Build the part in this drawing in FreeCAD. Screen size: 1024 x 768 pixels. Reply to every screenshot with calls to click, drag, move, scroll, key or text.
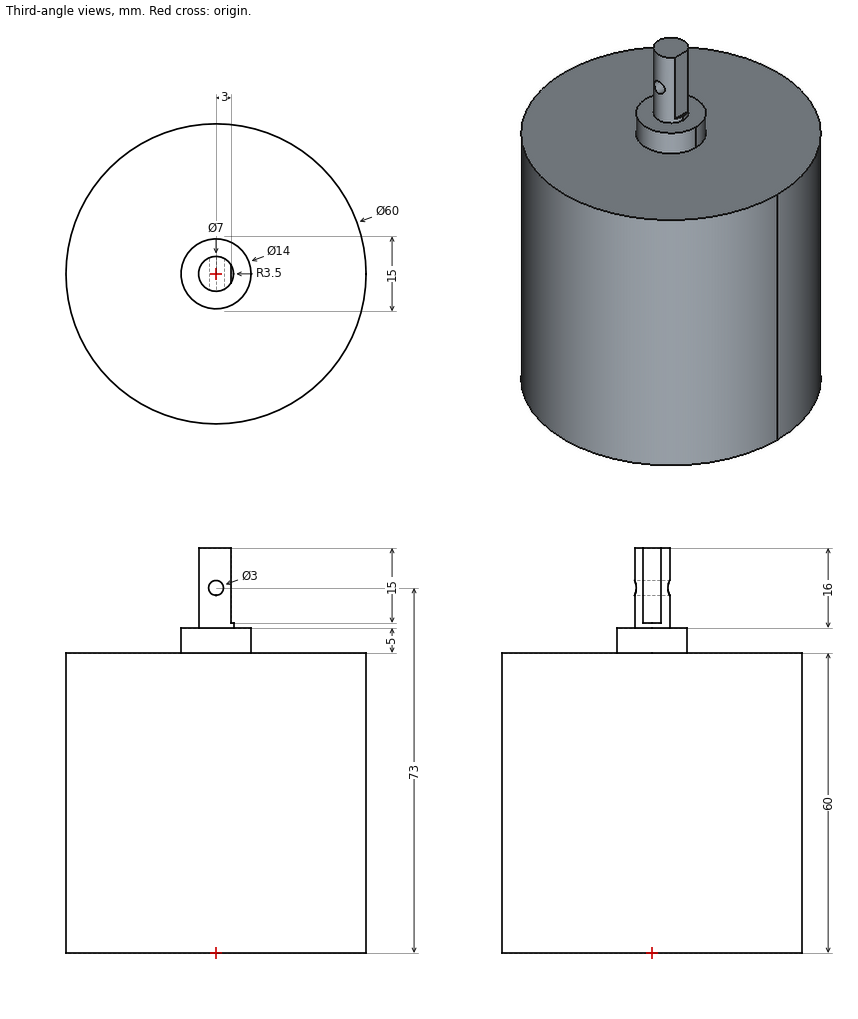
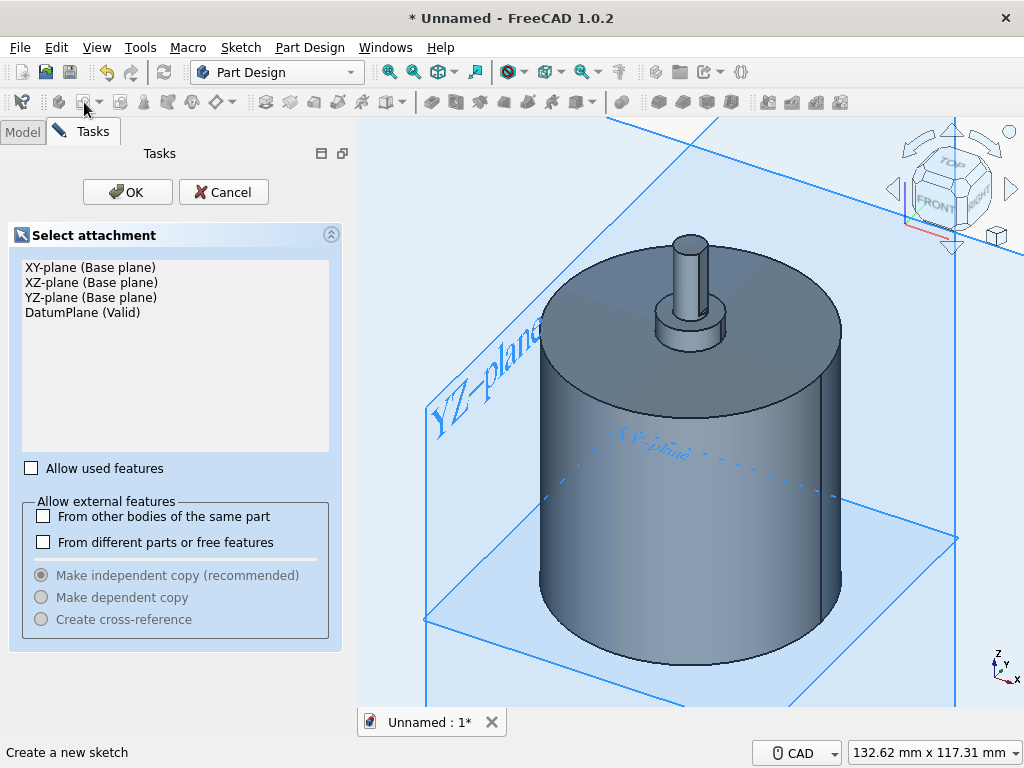
click(82, 282)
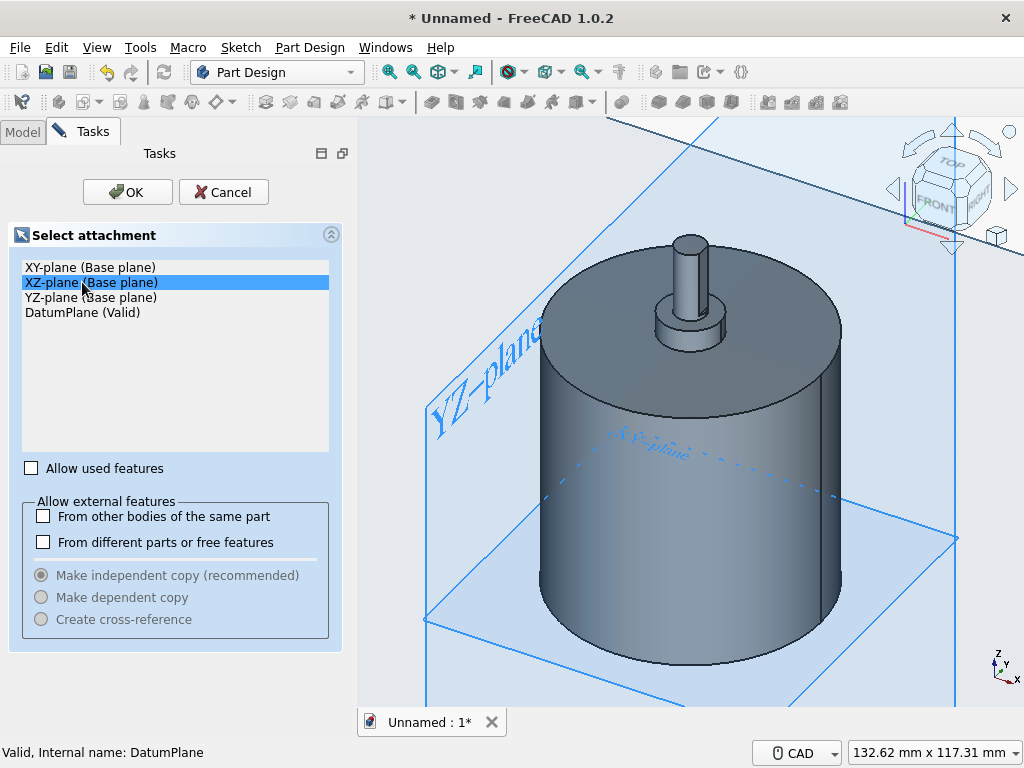
click(128, 192)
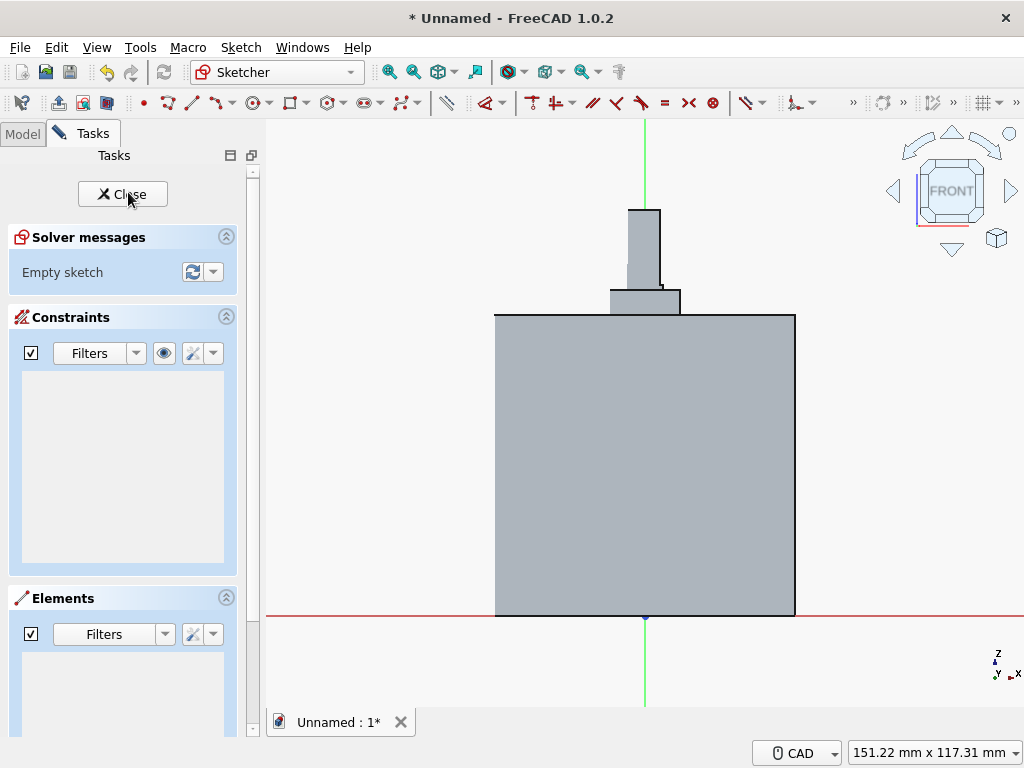
click(108, 104)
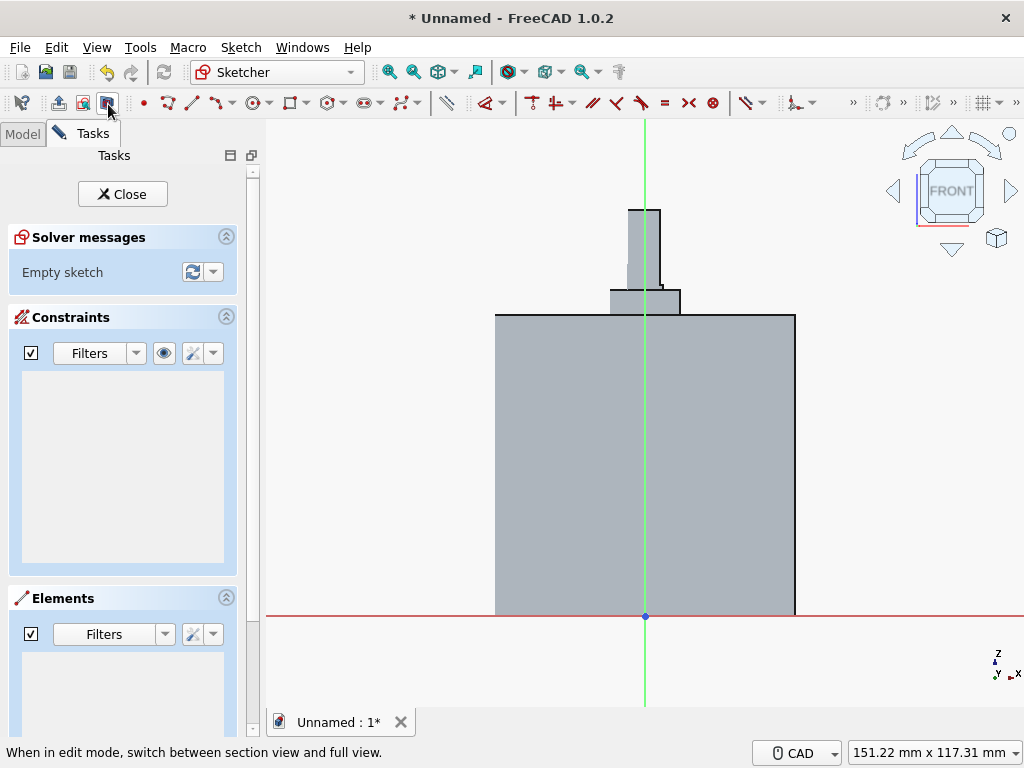
scroll(649, 242, up, 15)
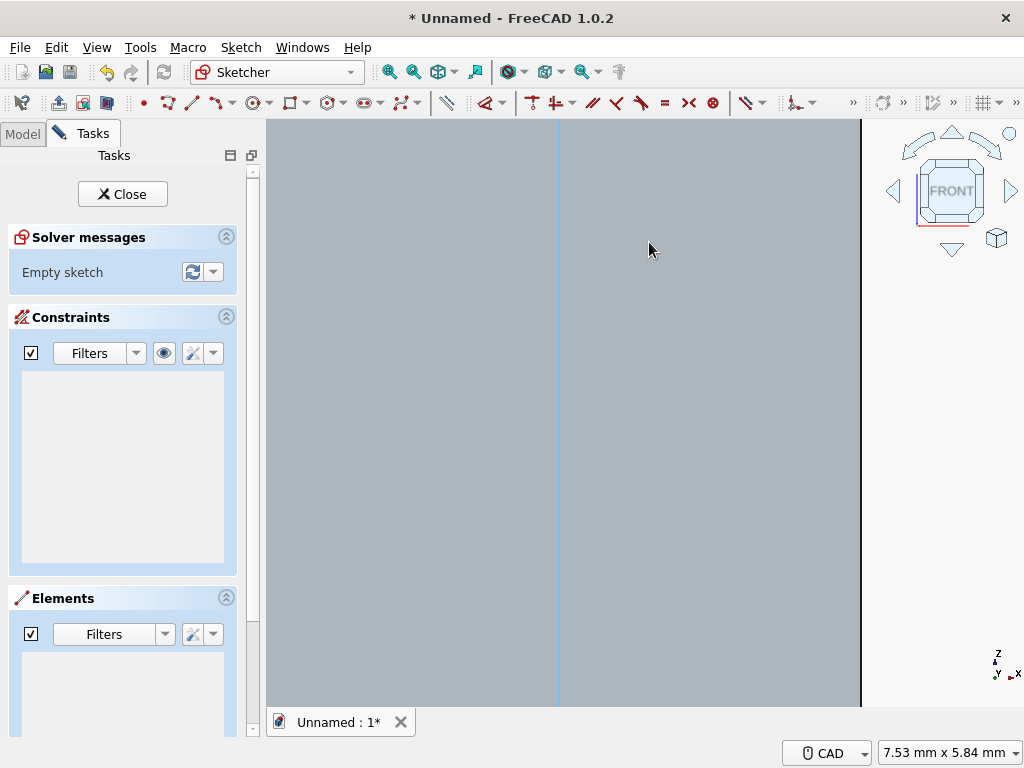
click(254, 104)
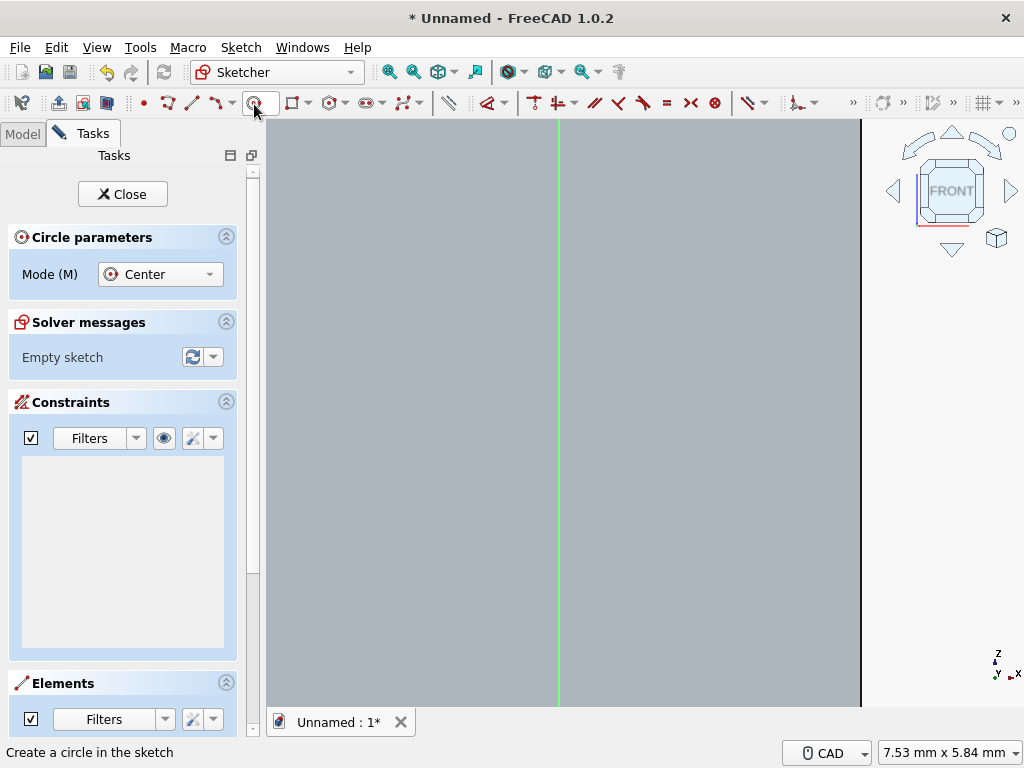
click(559, 401)
move(666, 294)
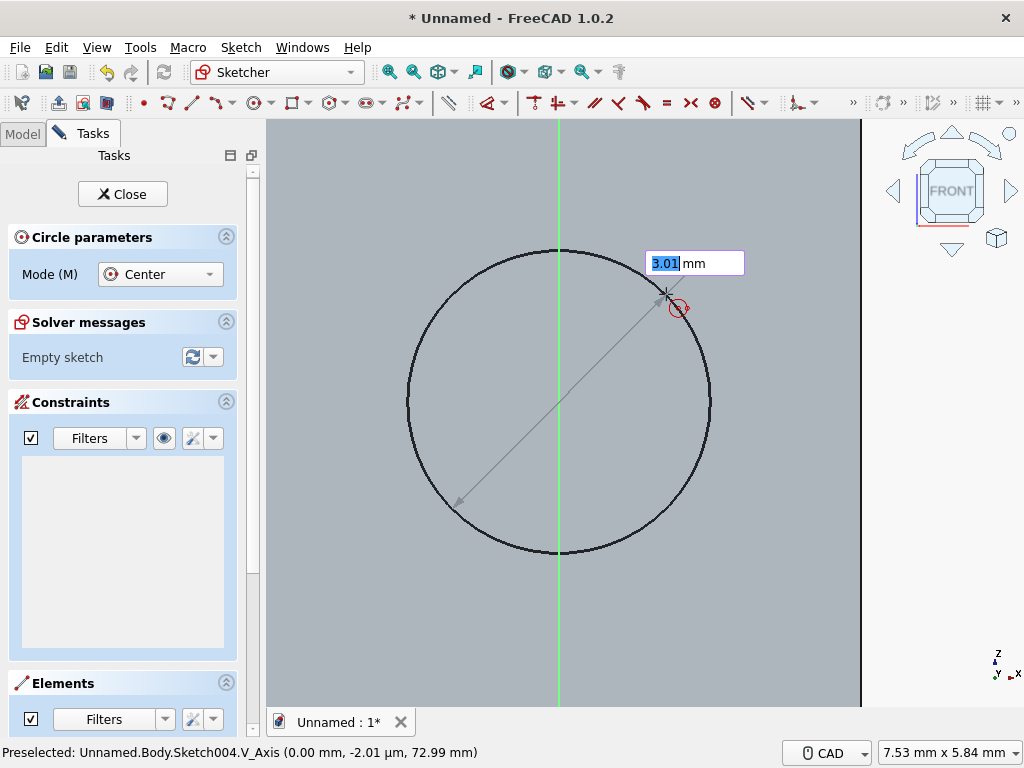
text(3)
key(Return)
key(Escape)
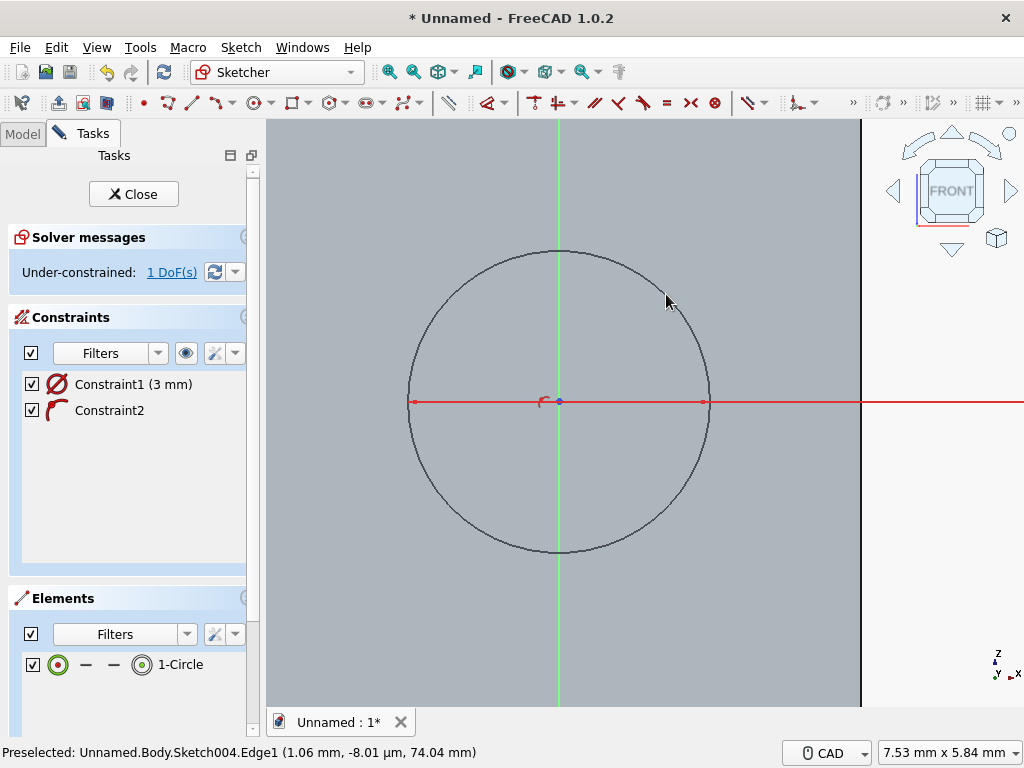
click(488, 104)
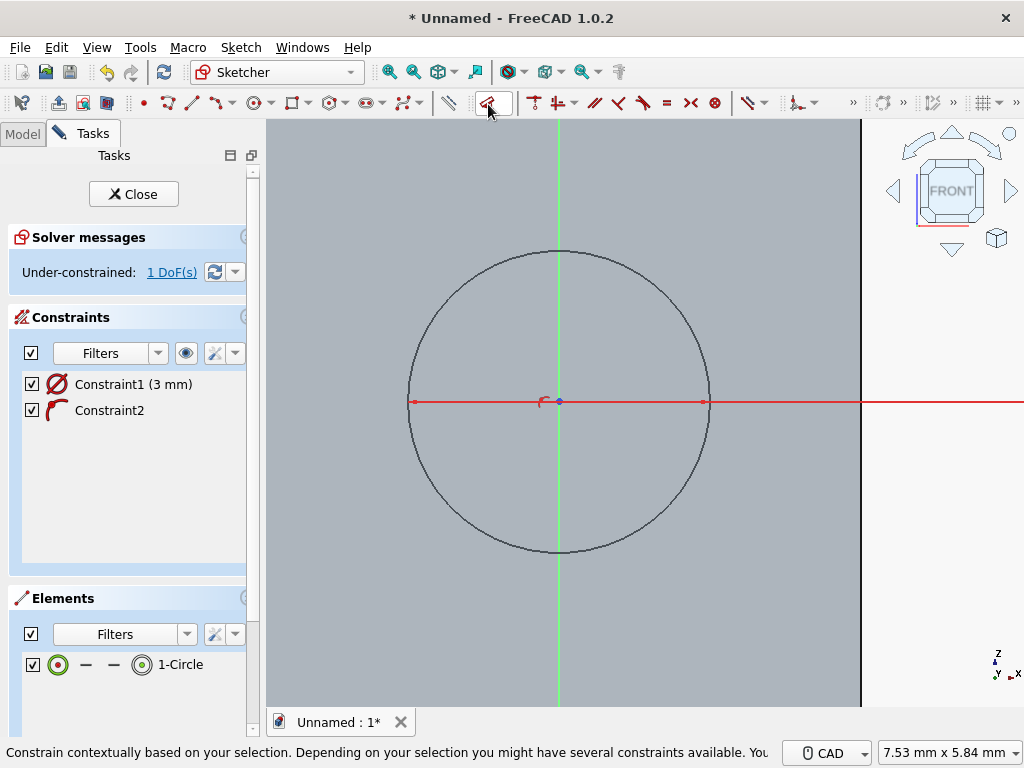
click(559, 402)
click(593, 477)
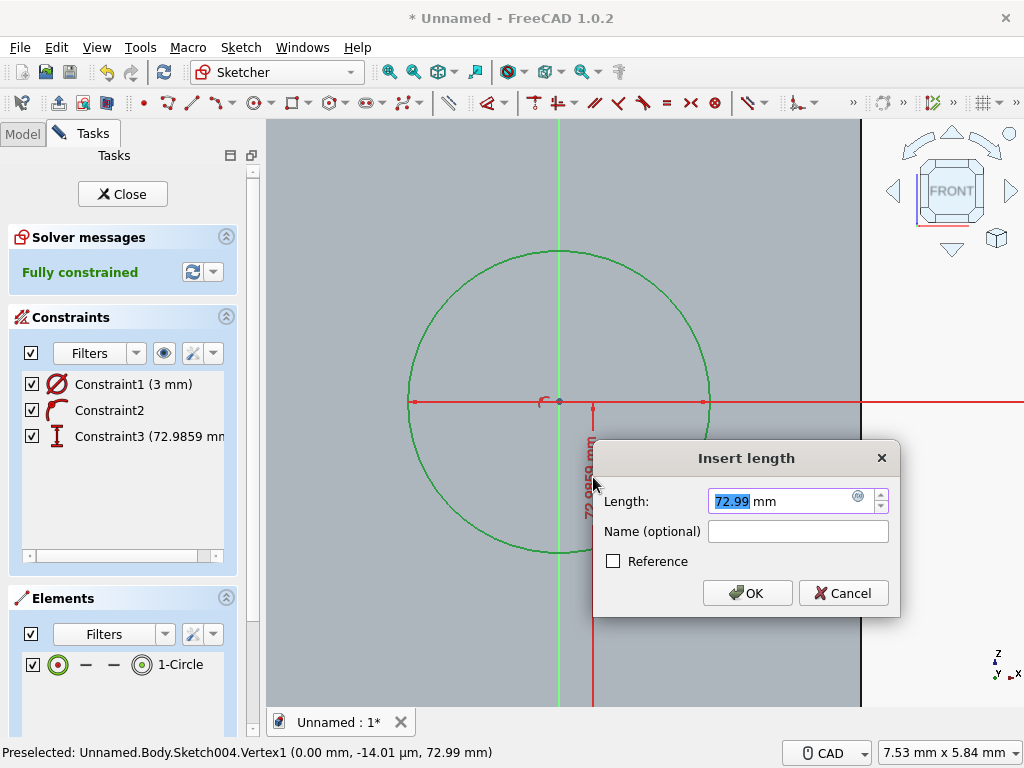
text(73)
key(Return)
key(Escape)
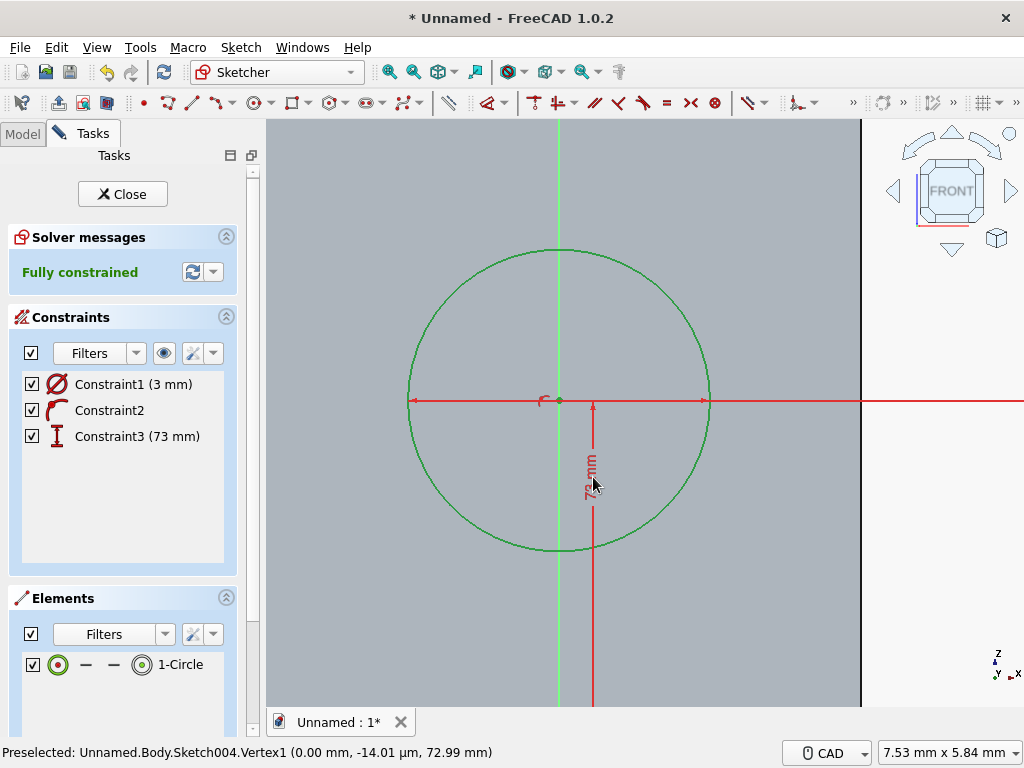
click(123, 194)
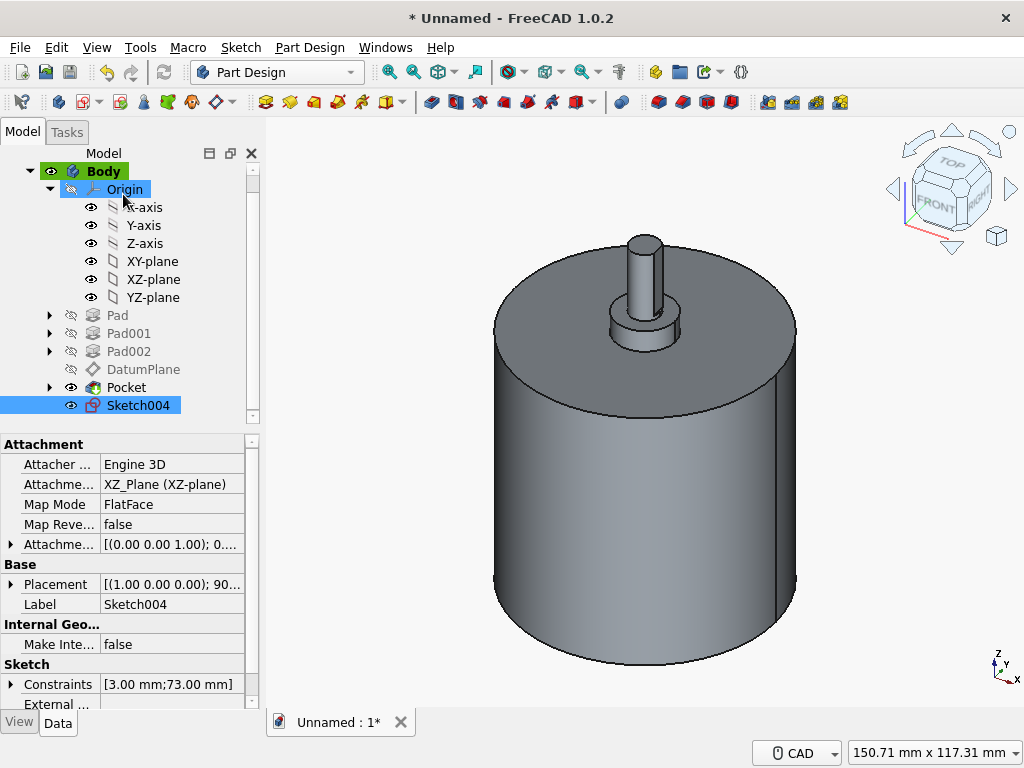
click(432, 102)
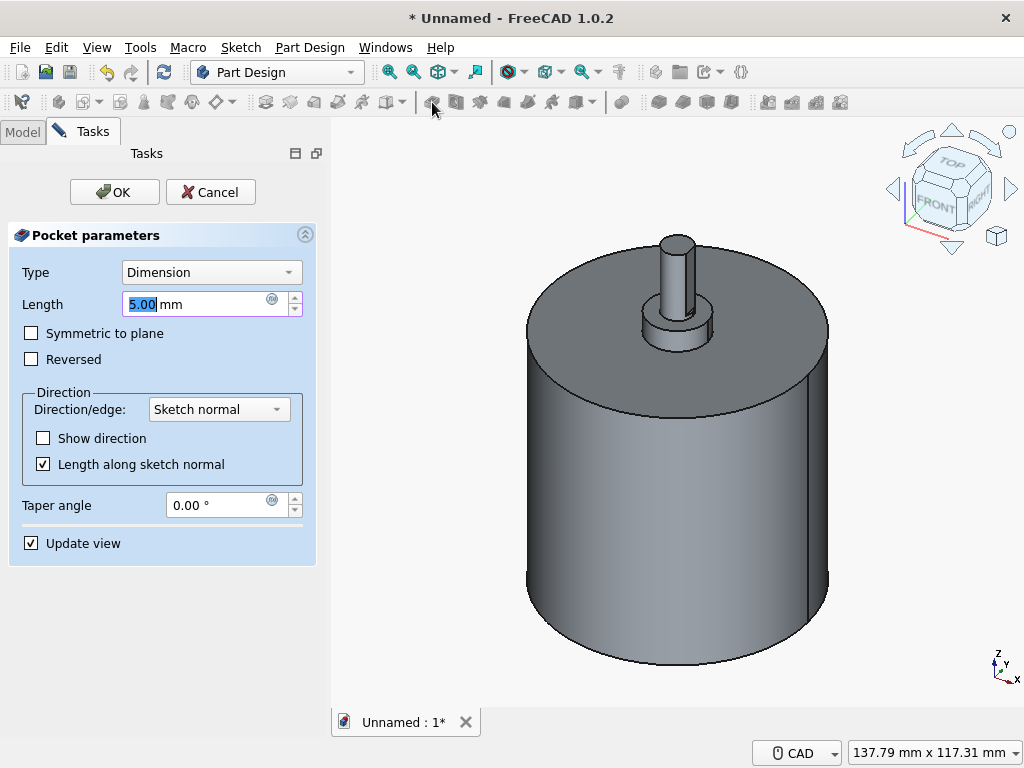
text(15)
key(Tab)